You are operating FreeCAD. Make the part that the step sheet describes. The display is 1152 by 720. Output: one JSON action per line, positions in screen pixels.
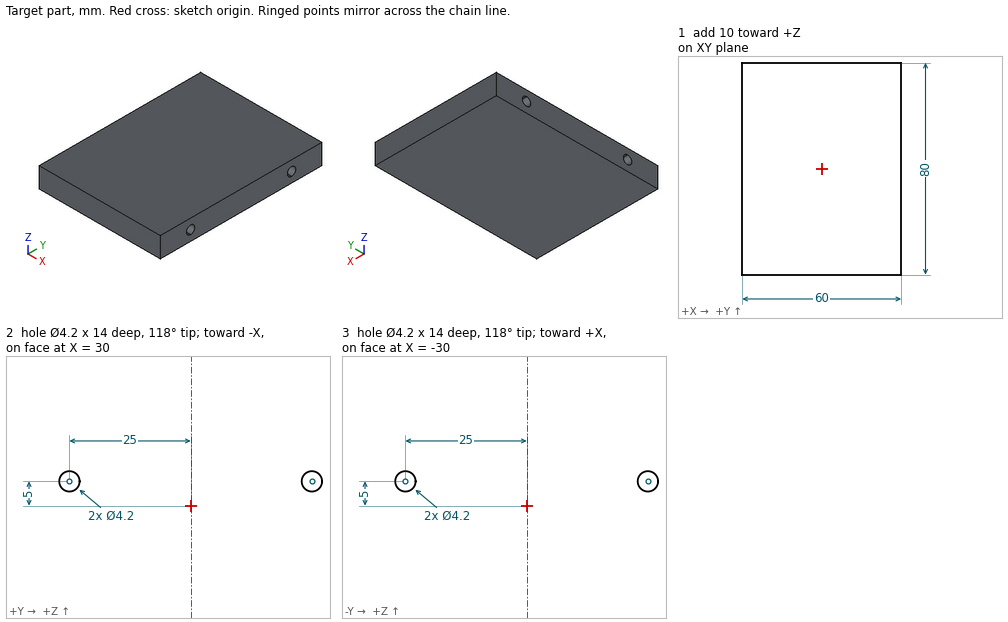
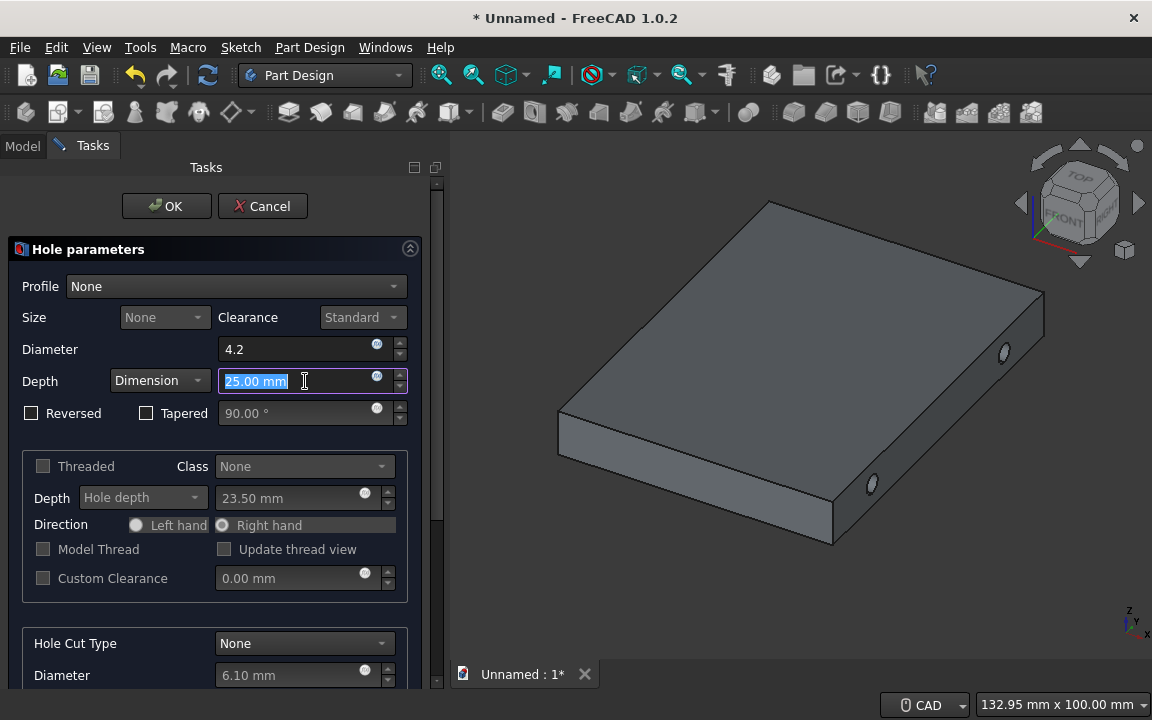
{"action": "type", "text": "14"}
{"action": "key", "text": "Tab"}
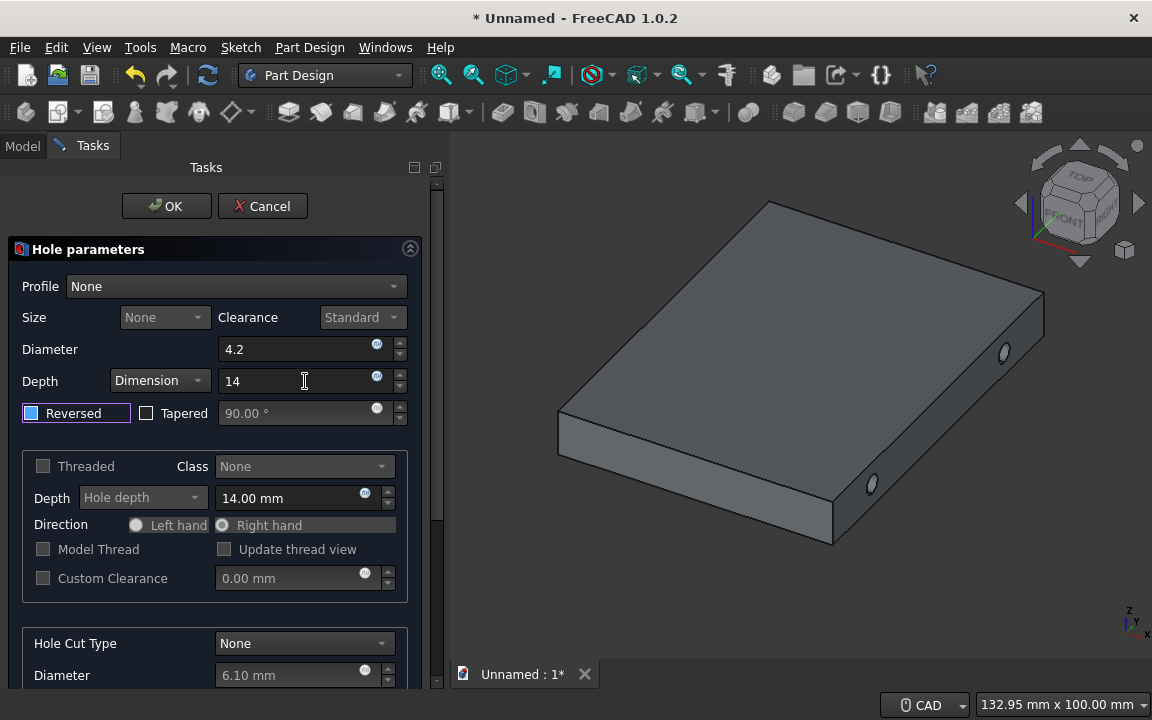
{"action": "left_click", "coordinate": [167, 206]}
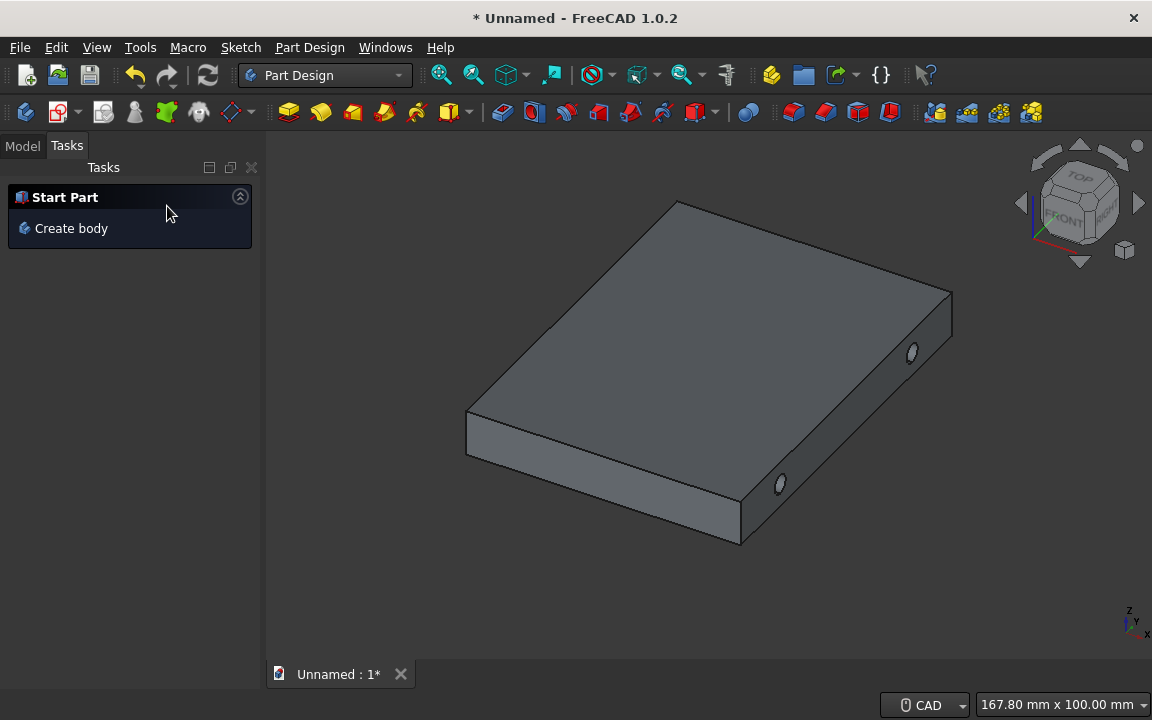
{"action": "key", "text": "6"}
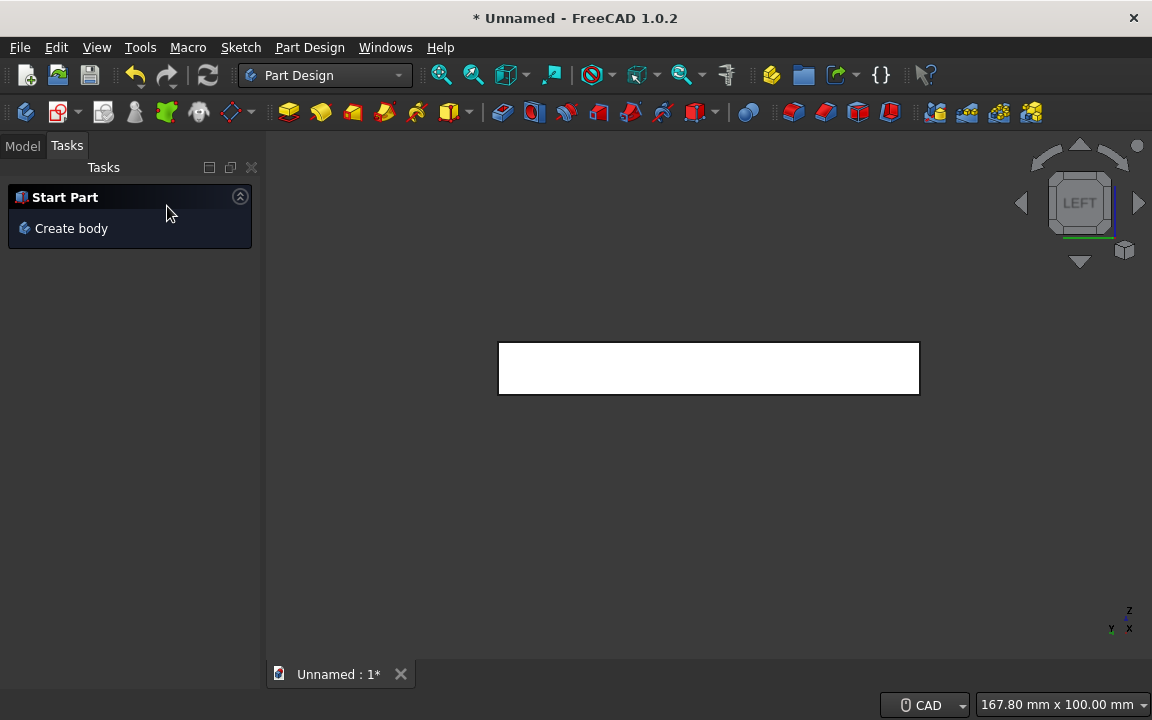
{"action": "left_click", "coordinate": [528, 368]}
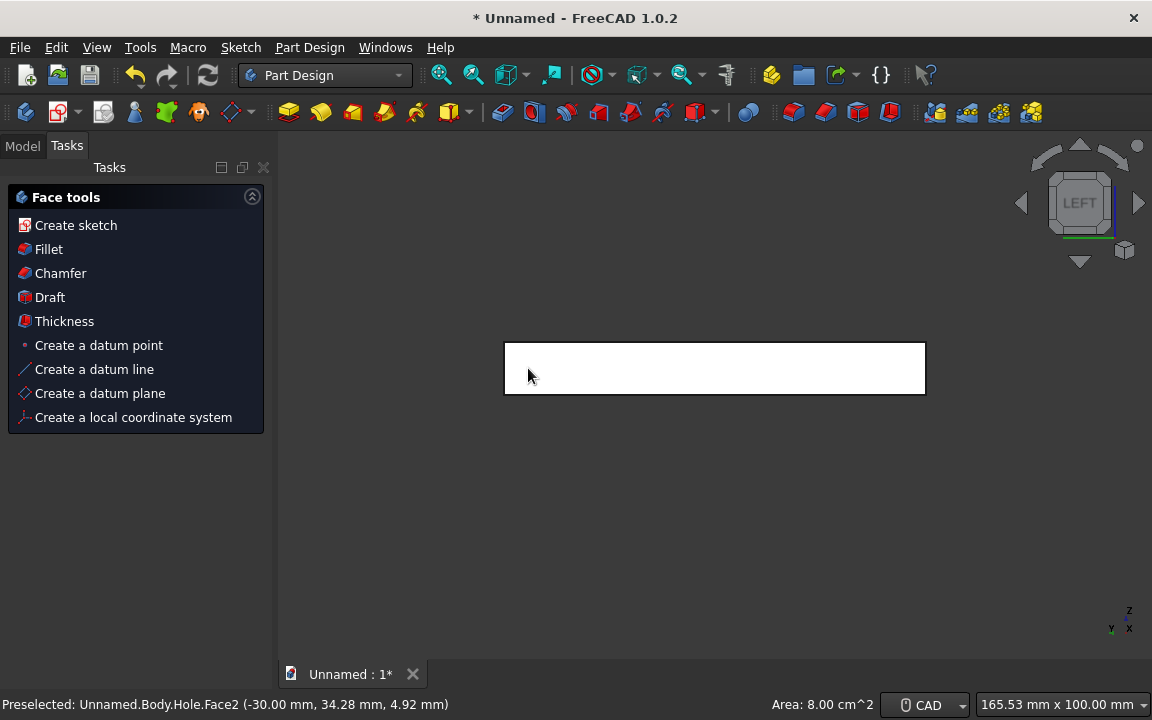
{"action": "left_click", "coordinate": [58, 112]}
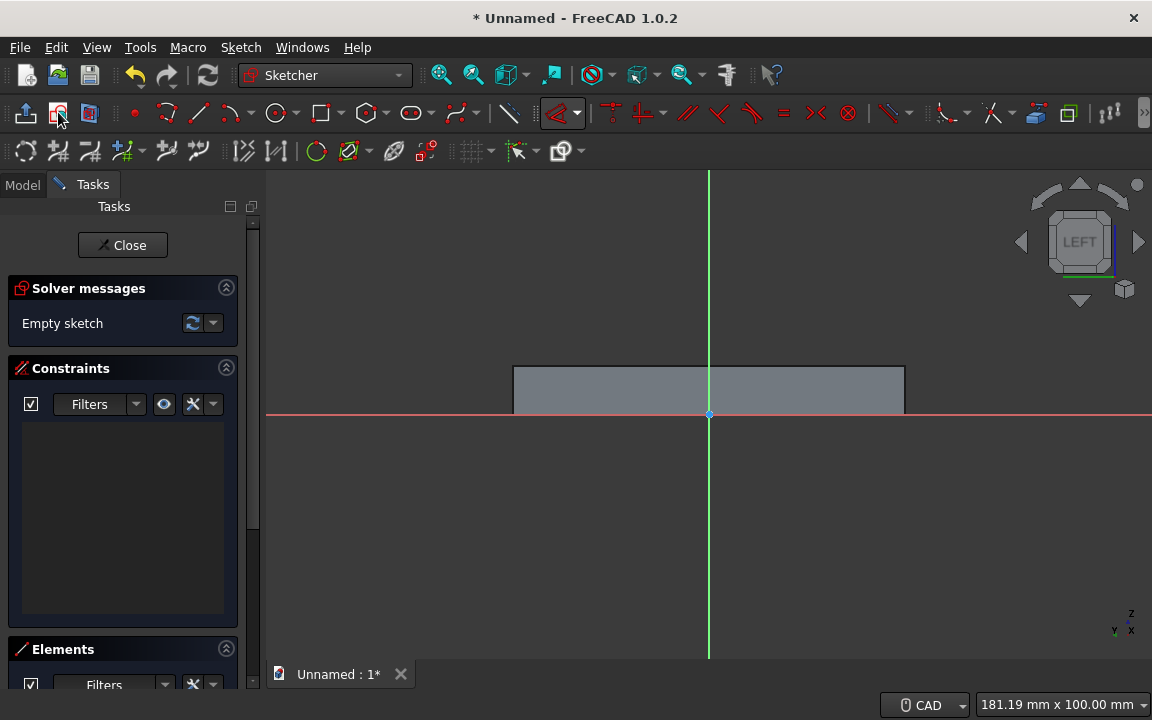
{"action": "scroll", "coordinate": [792, 376], "scroll_direction": "up", "scroll_amount": 3}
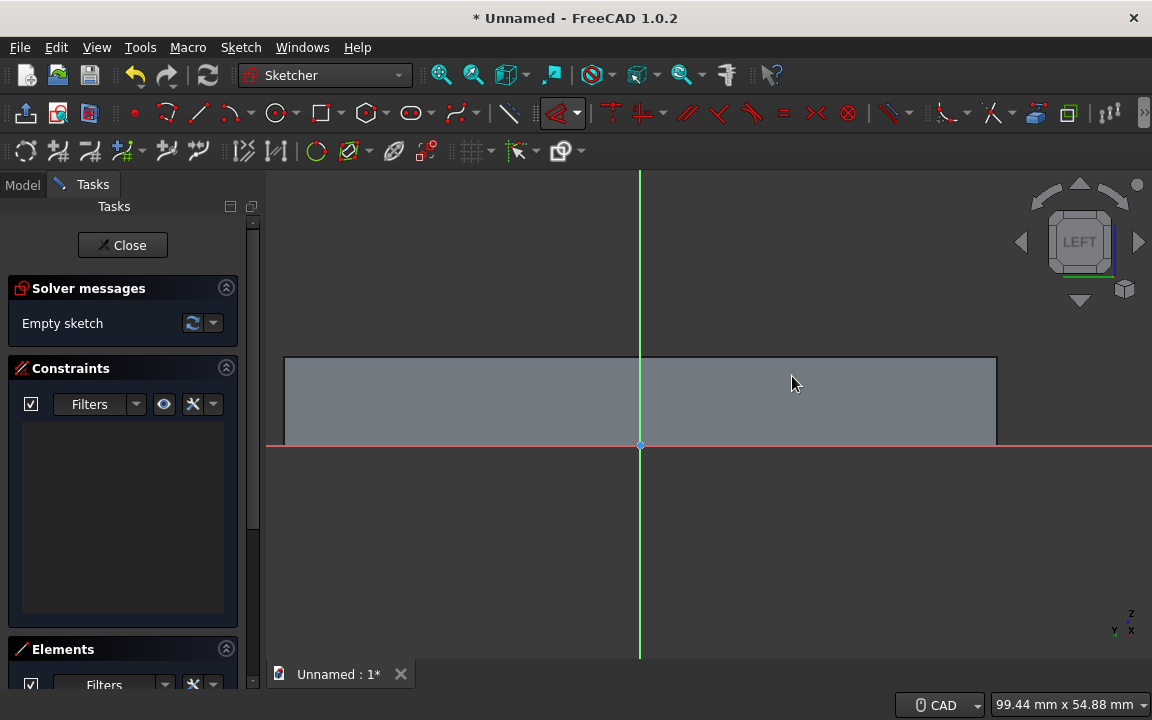
{"action": "left_click", "coordinate": [276, 114]}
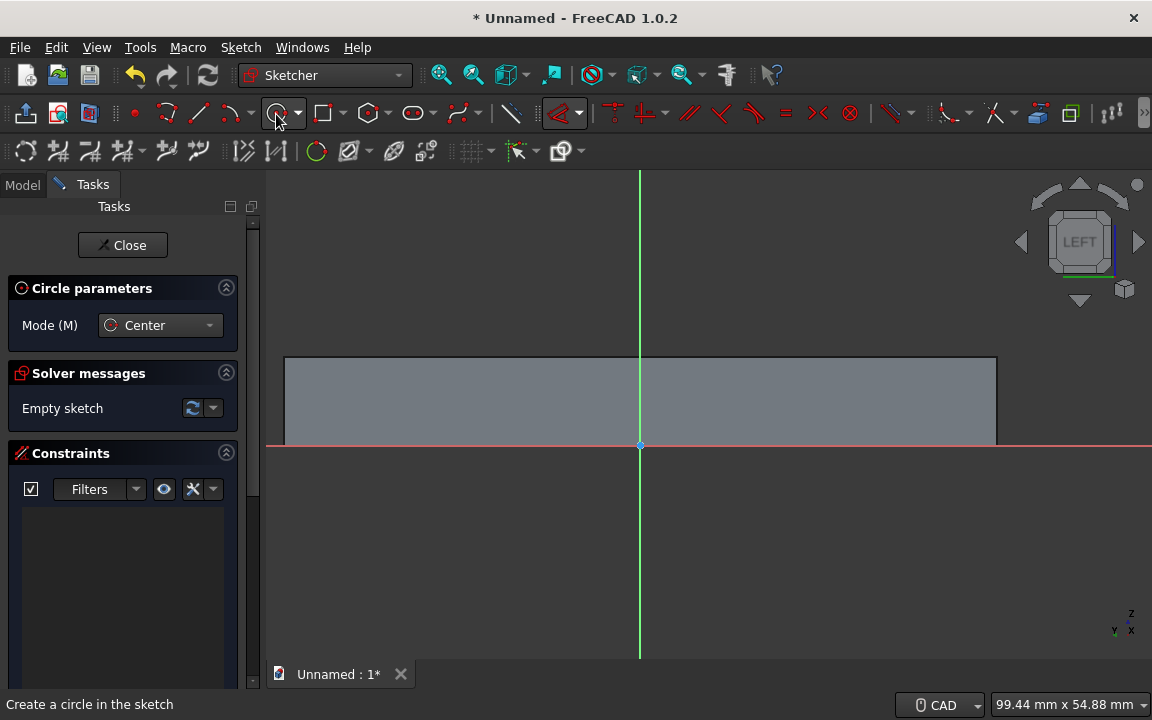
{"action": "left_click", "coordinate": [418, 401]}
{"action": "mouse_move", "coordinate": [431, 388]}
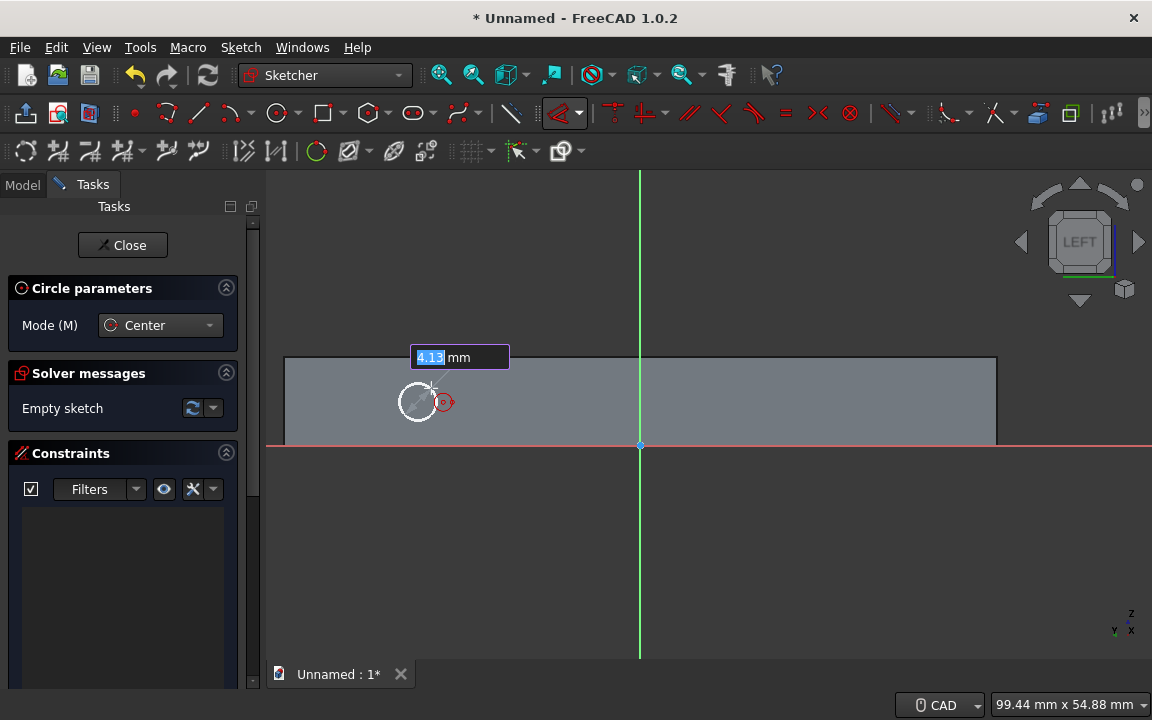
{"action": "type", "text": "4.2"}
{"action": "key", "text": "Return"}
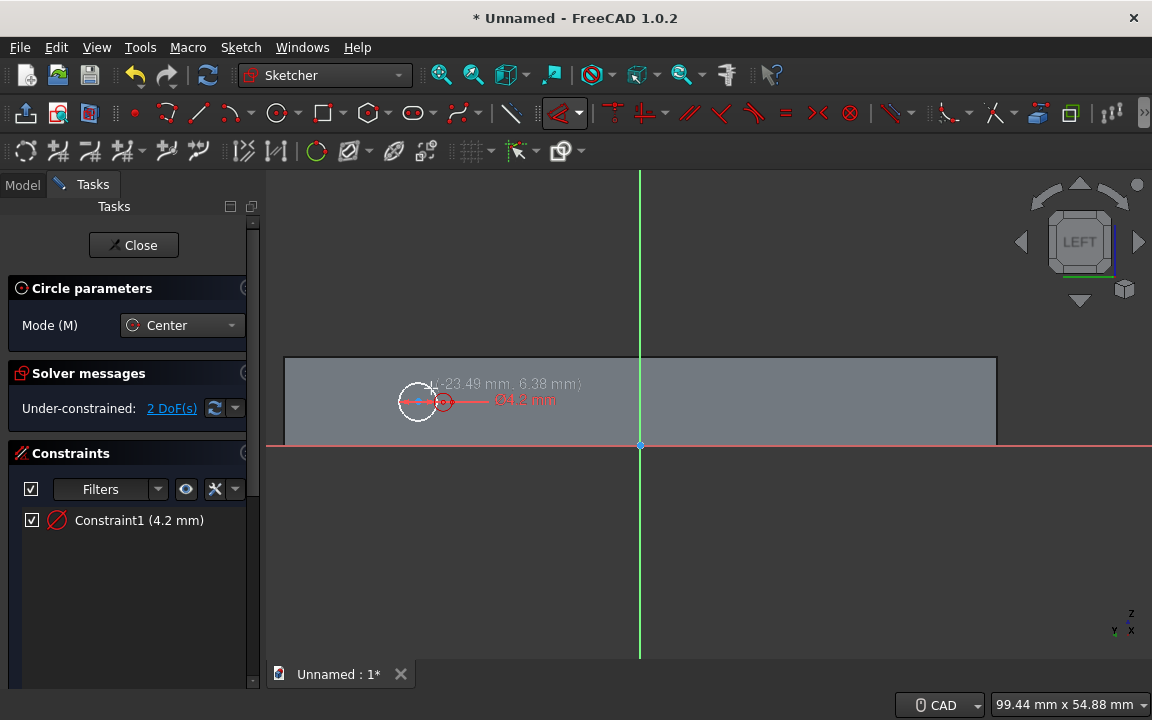
{"action": "left_click", "coordinate": [863, 401]}
{"action": "mouse_move", "coordinate": [876, 388]}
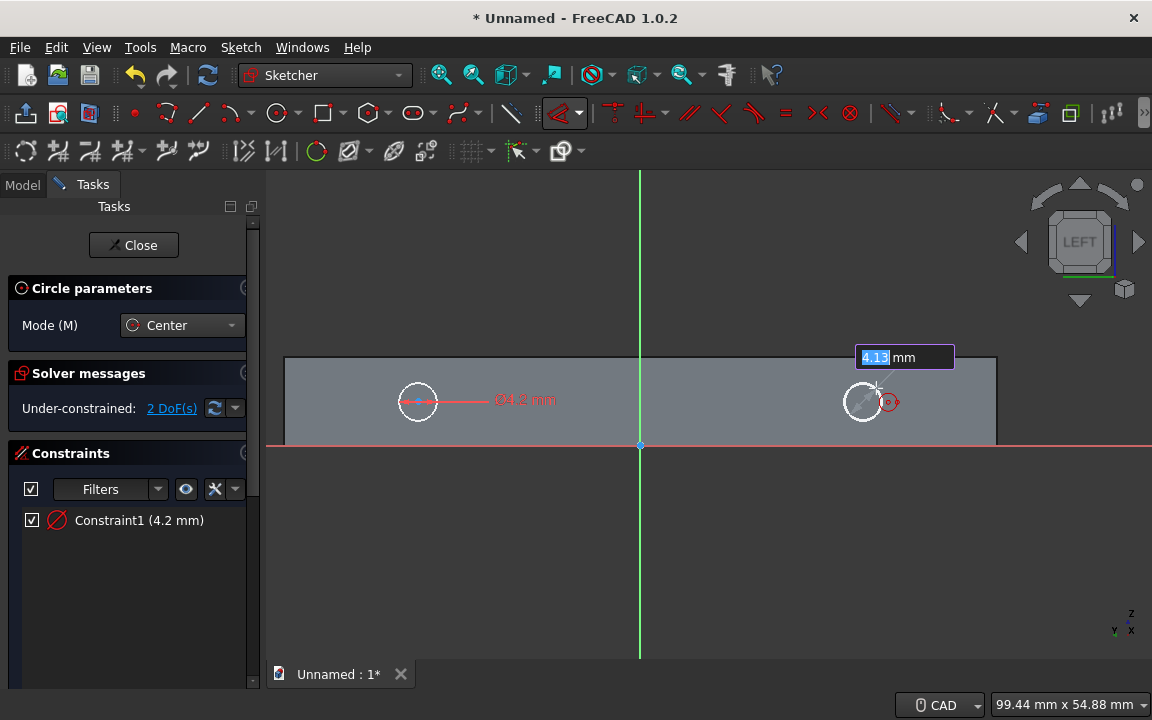
{"action": "type", "text": "4.2"}
{"action": "key", "text": "Return"}
{"action": "key", "text": "Escape"}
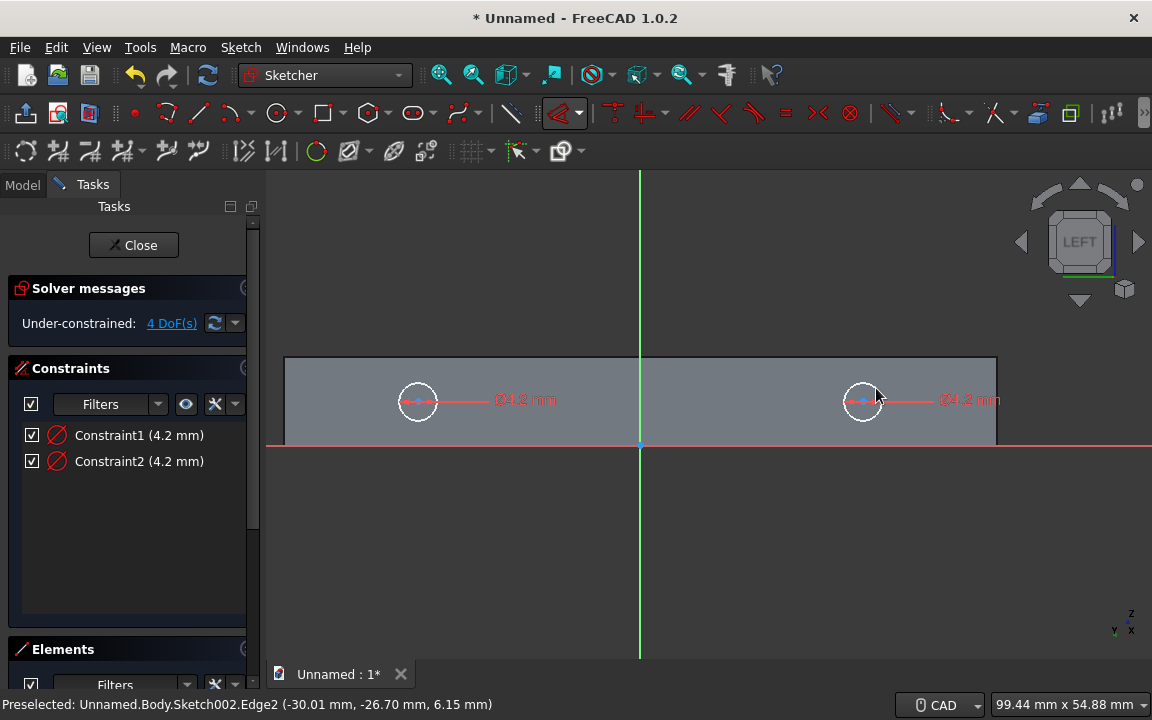
{"action": "left_click", "coordinate": [418, 402]}